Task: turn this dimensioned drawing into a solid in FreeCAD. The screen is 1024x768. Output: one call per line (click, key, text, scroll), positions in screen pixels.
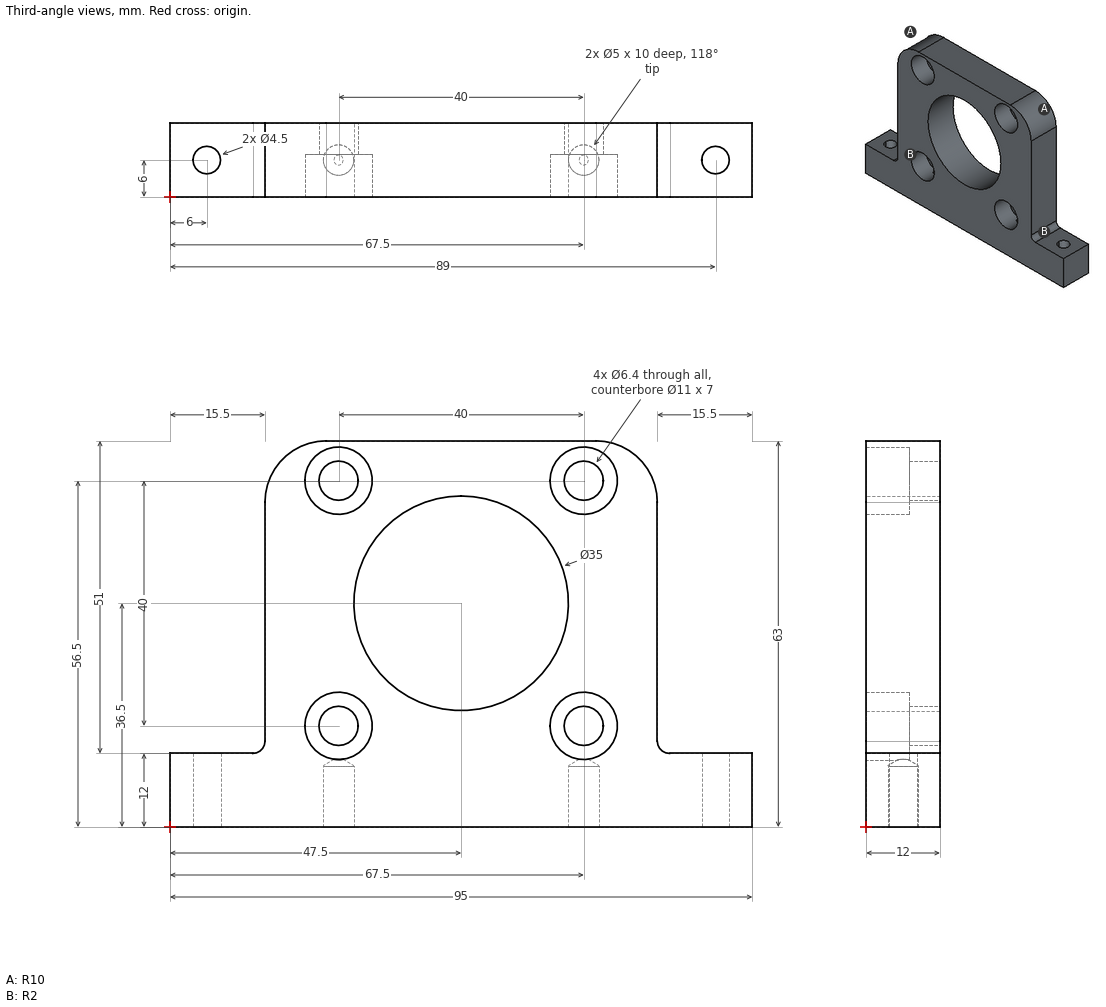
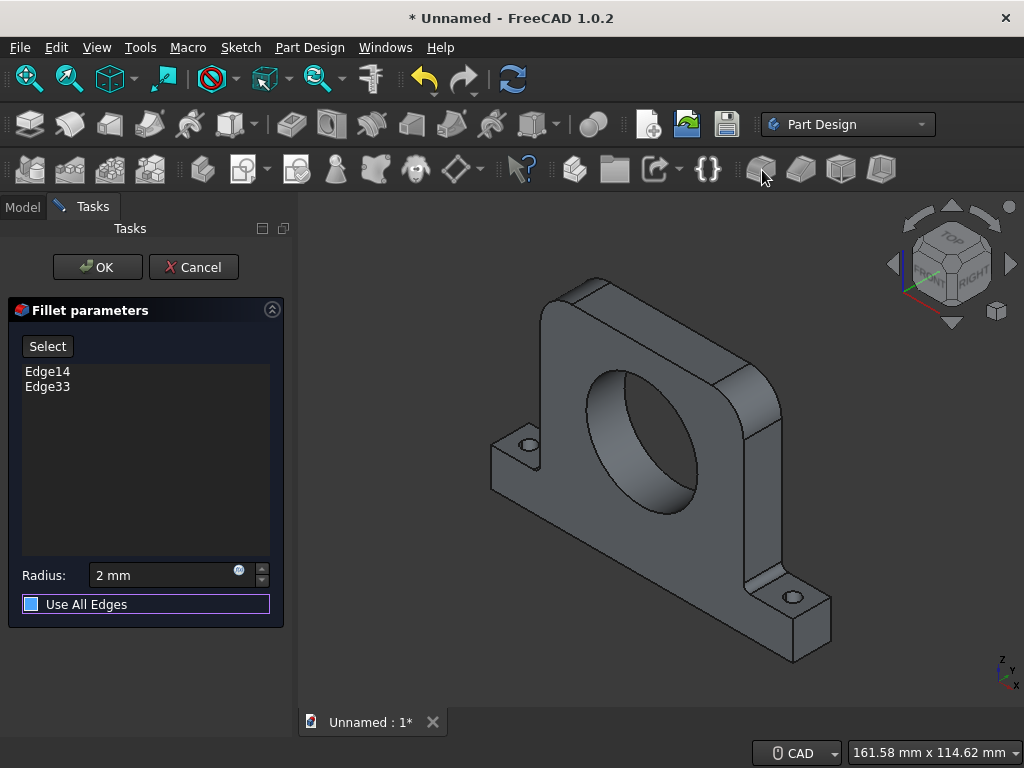
click(98, 267)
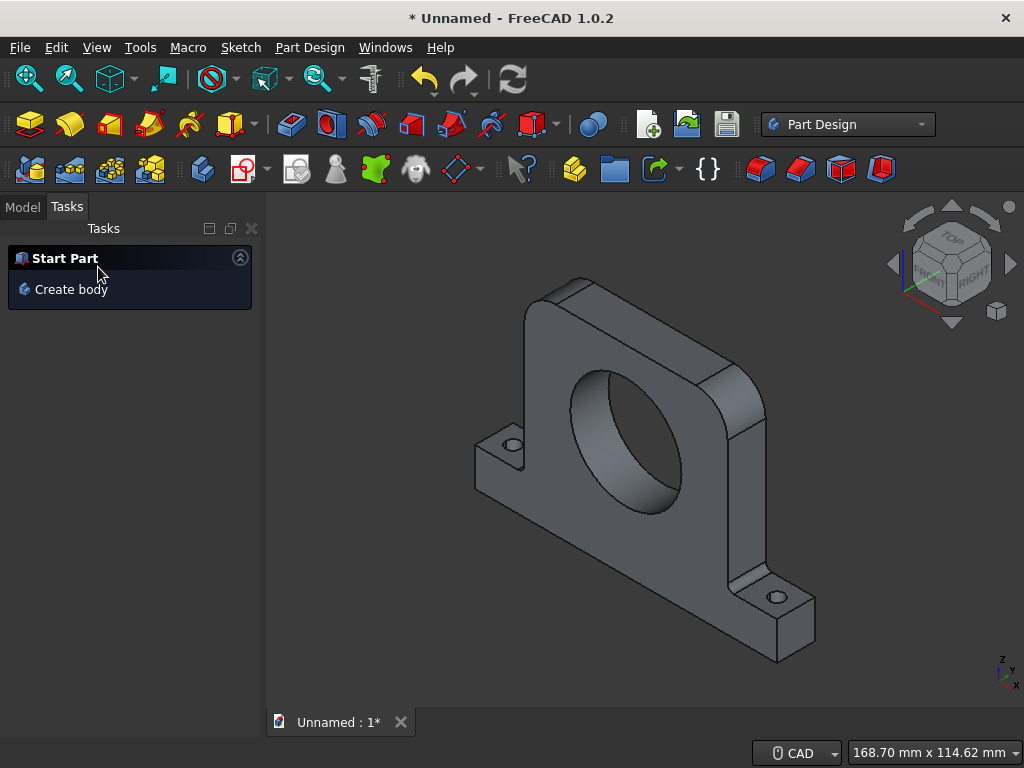
click(244, 170)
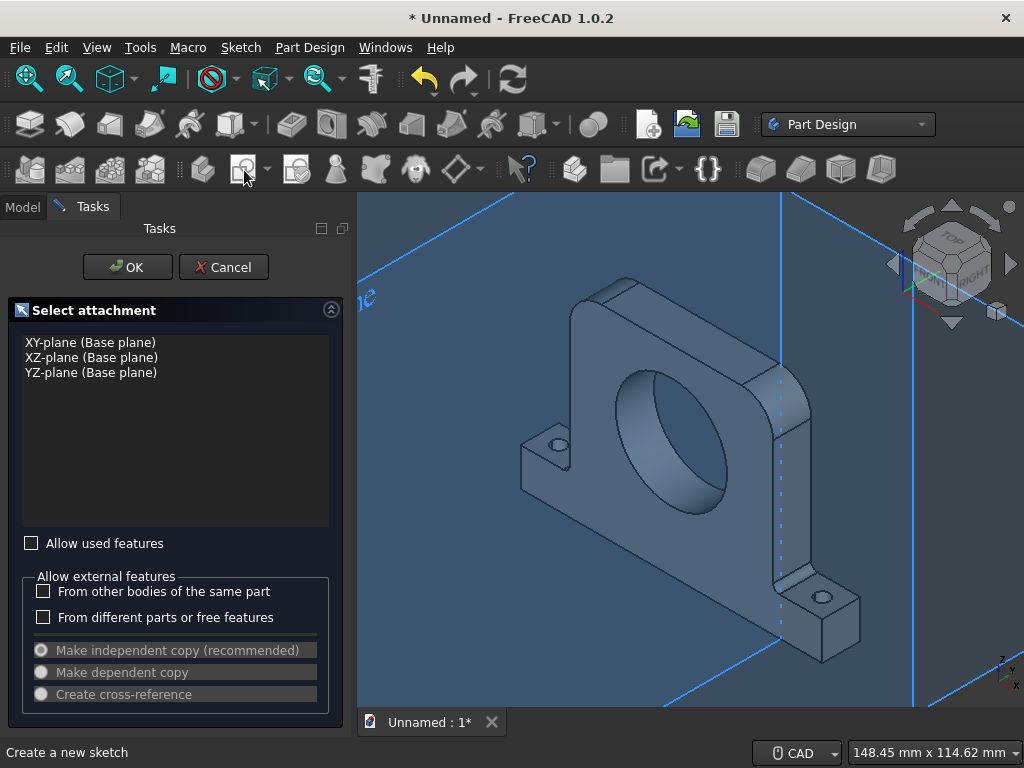
click(82, 358)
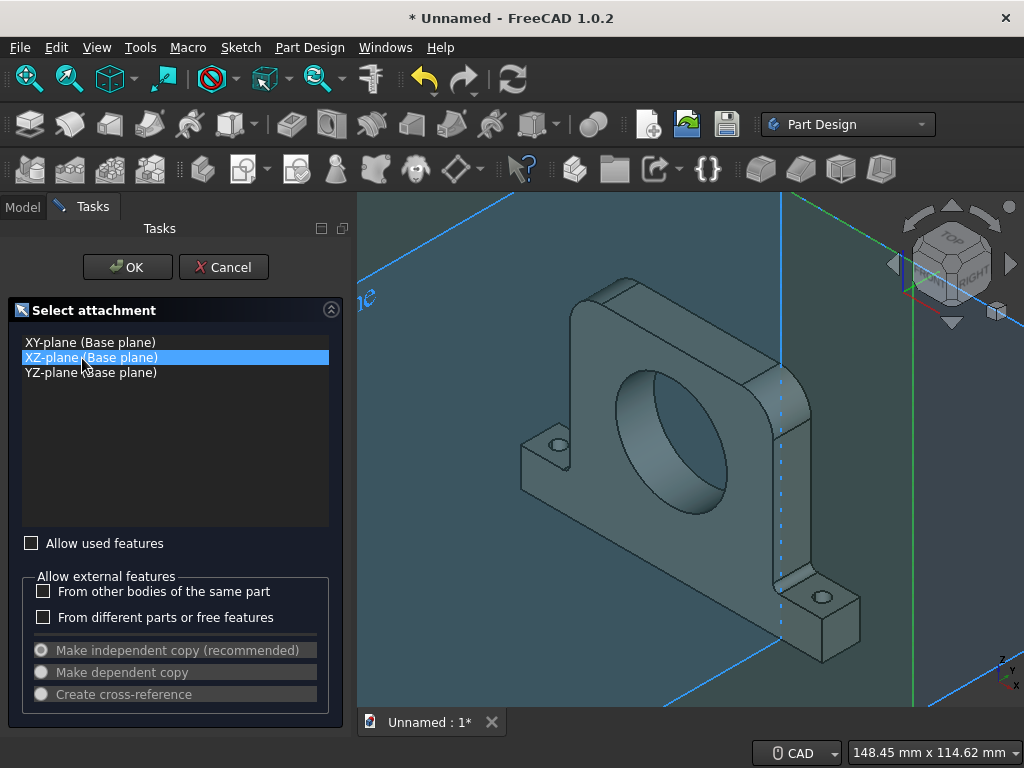
click(128, 267)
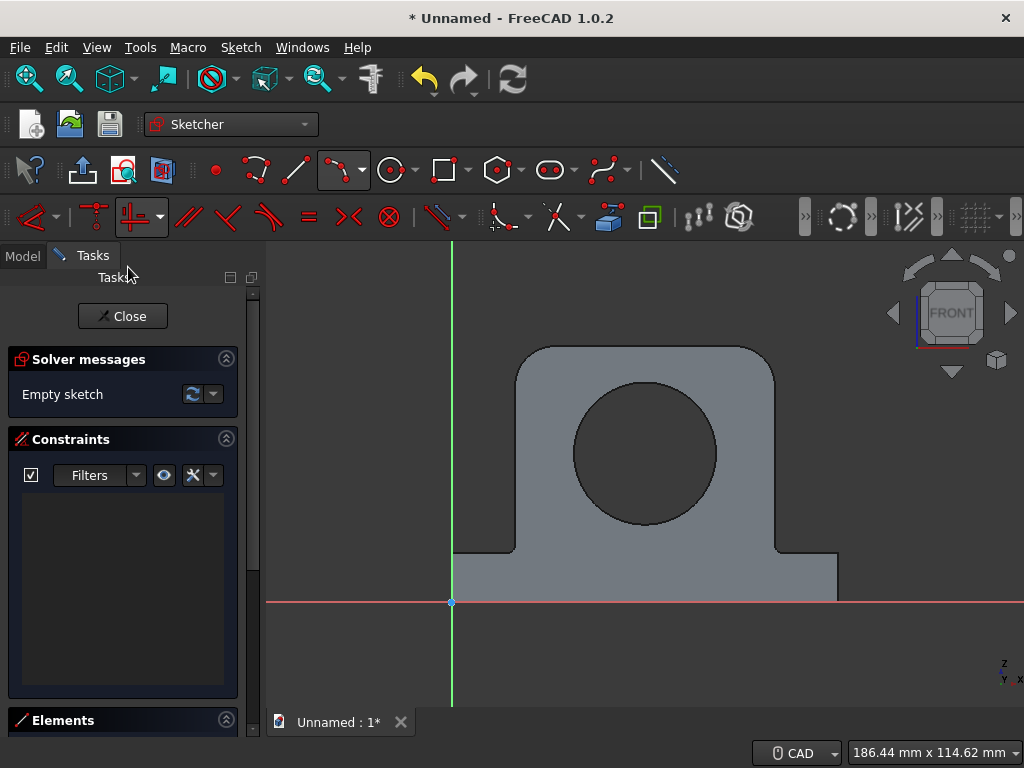
key(g)
key(c)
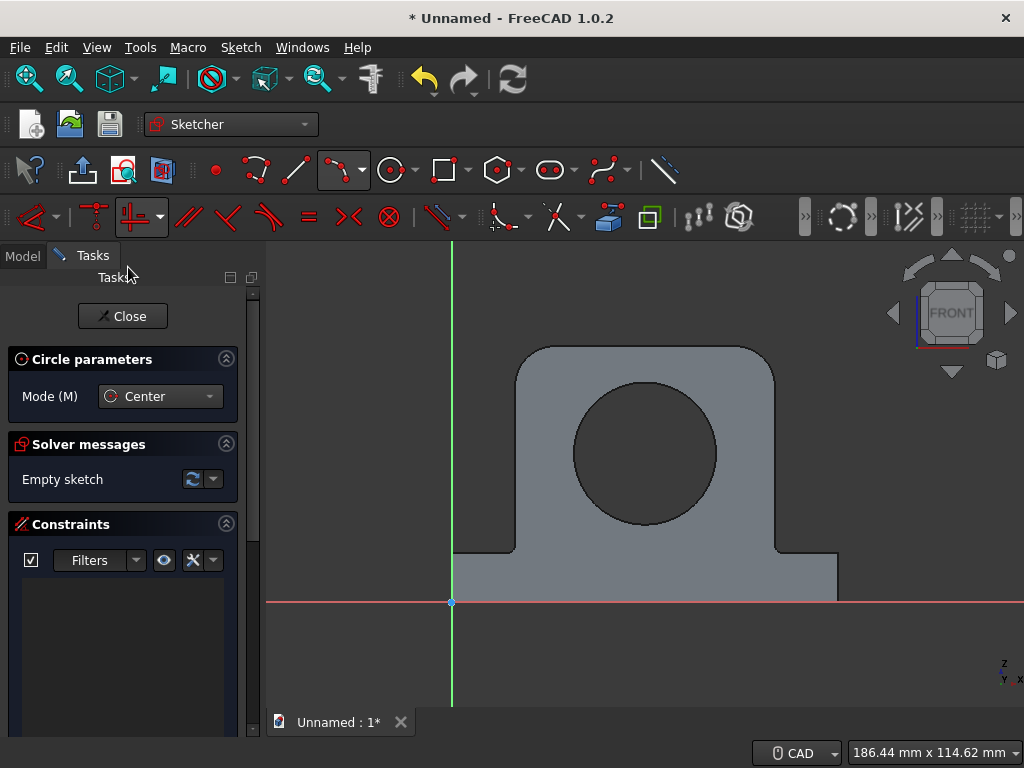
scroll(726, 372, up, 3)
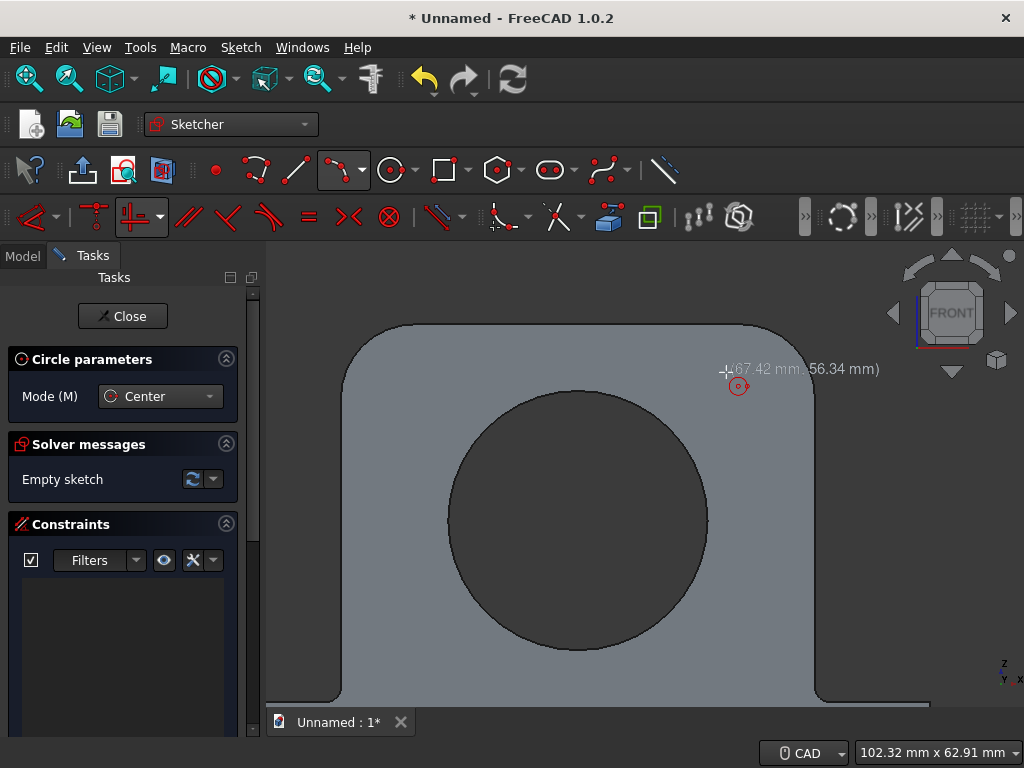
click(726, 372)
click(743, 356)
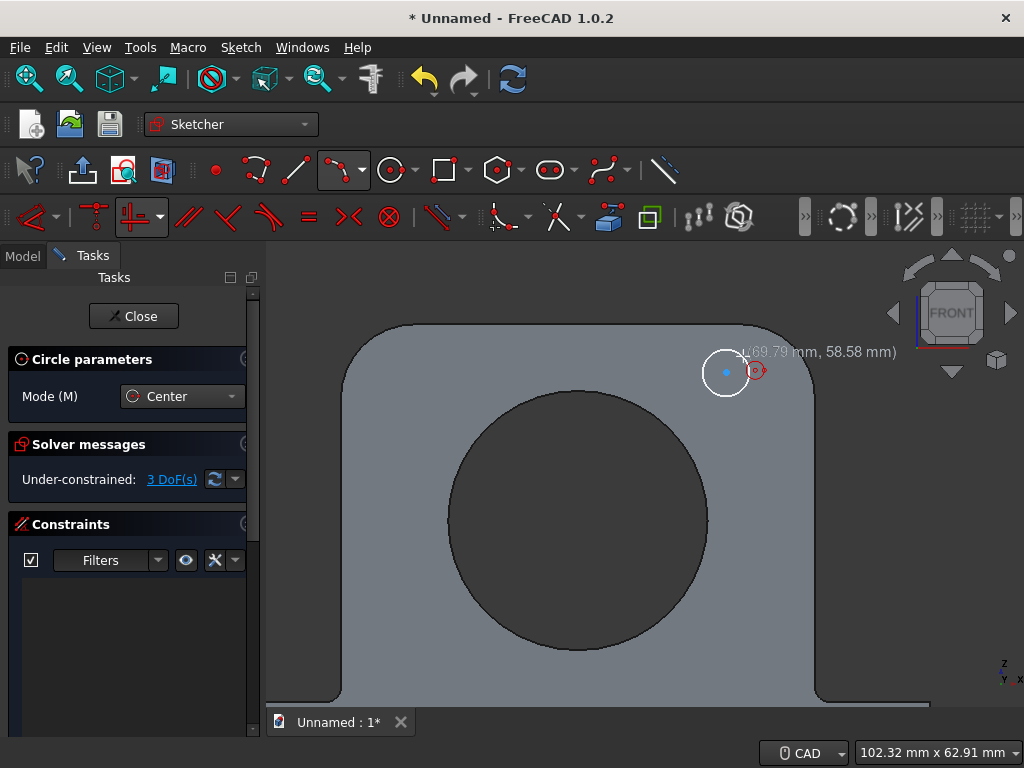
click(430, 372)
click(447, 356)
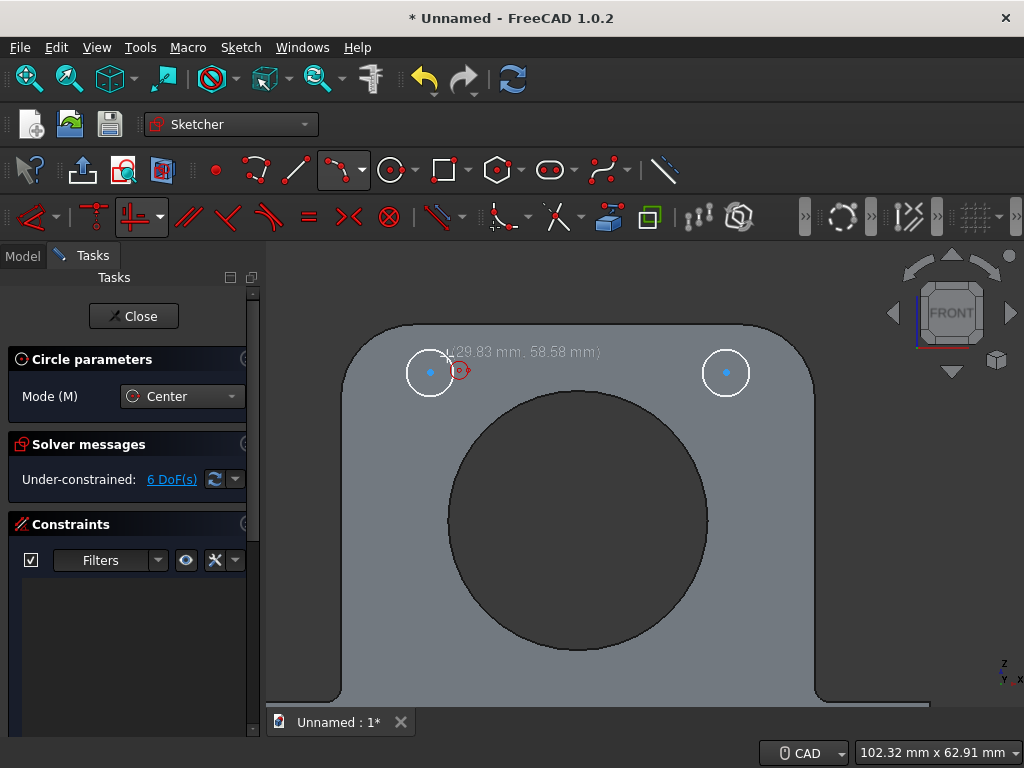
click(430, 669)
click(447, 652)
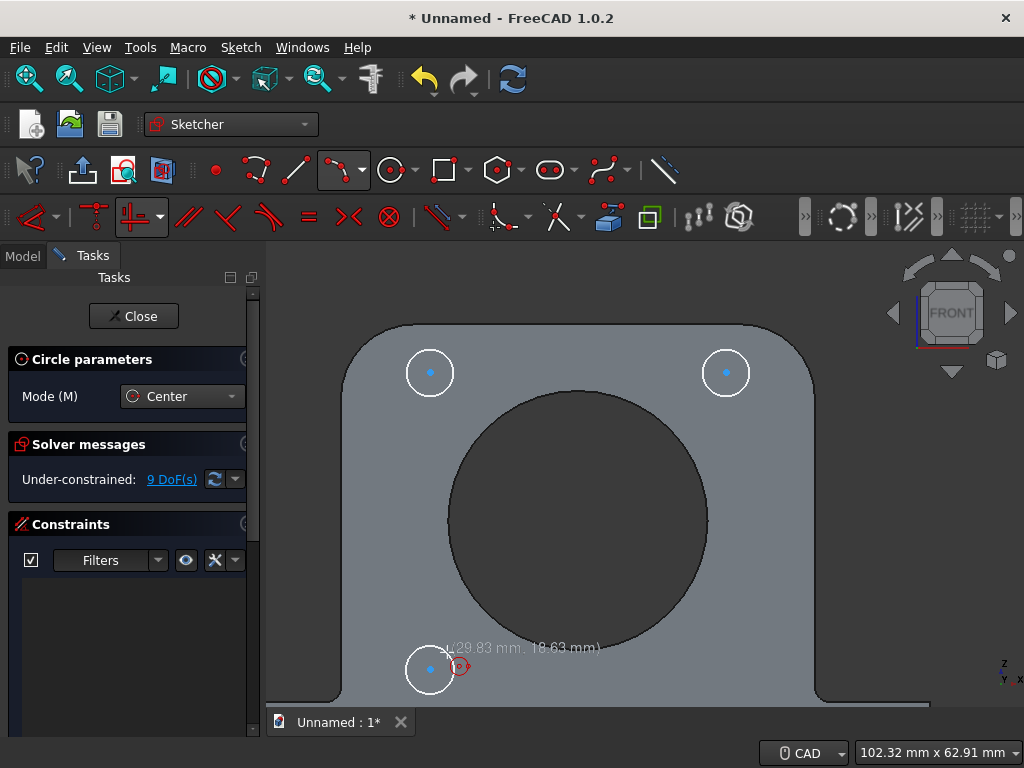
click(726, 669)
click(743, 652)
key(Escape)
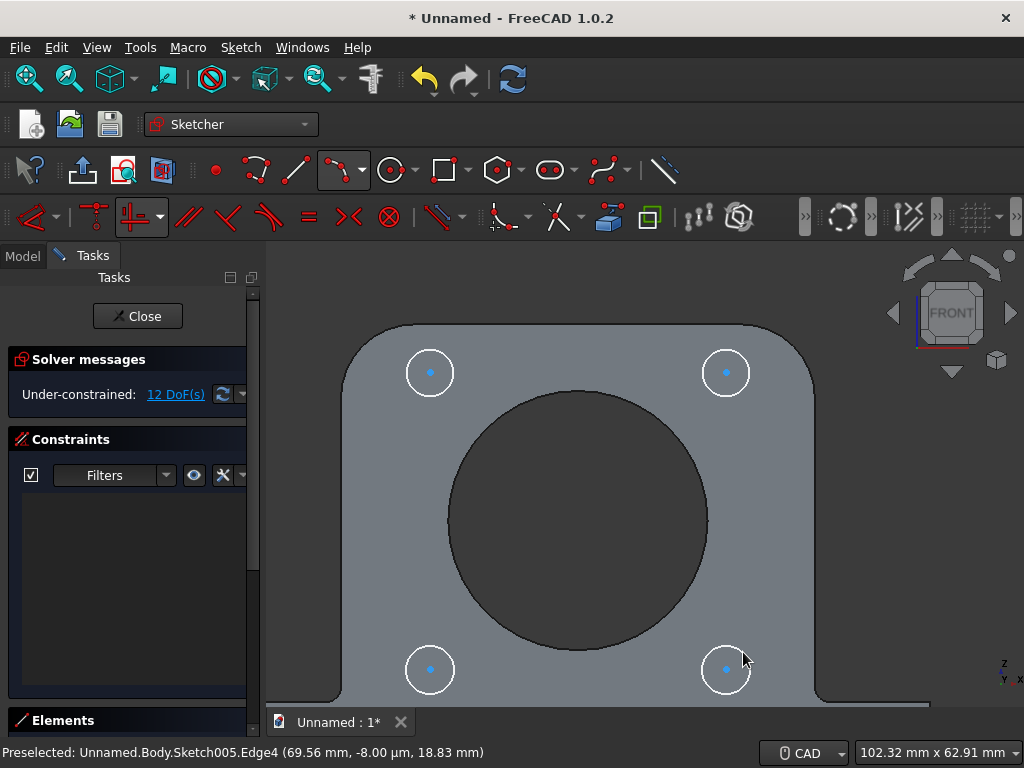
click(742, 356)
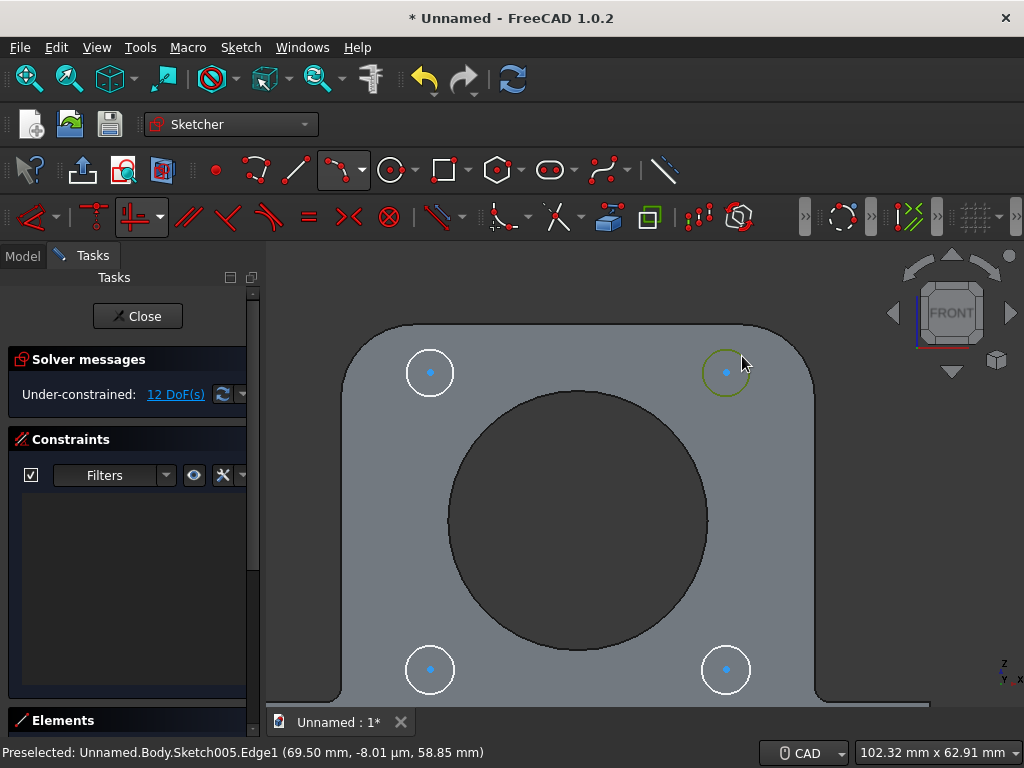
click(446, 356)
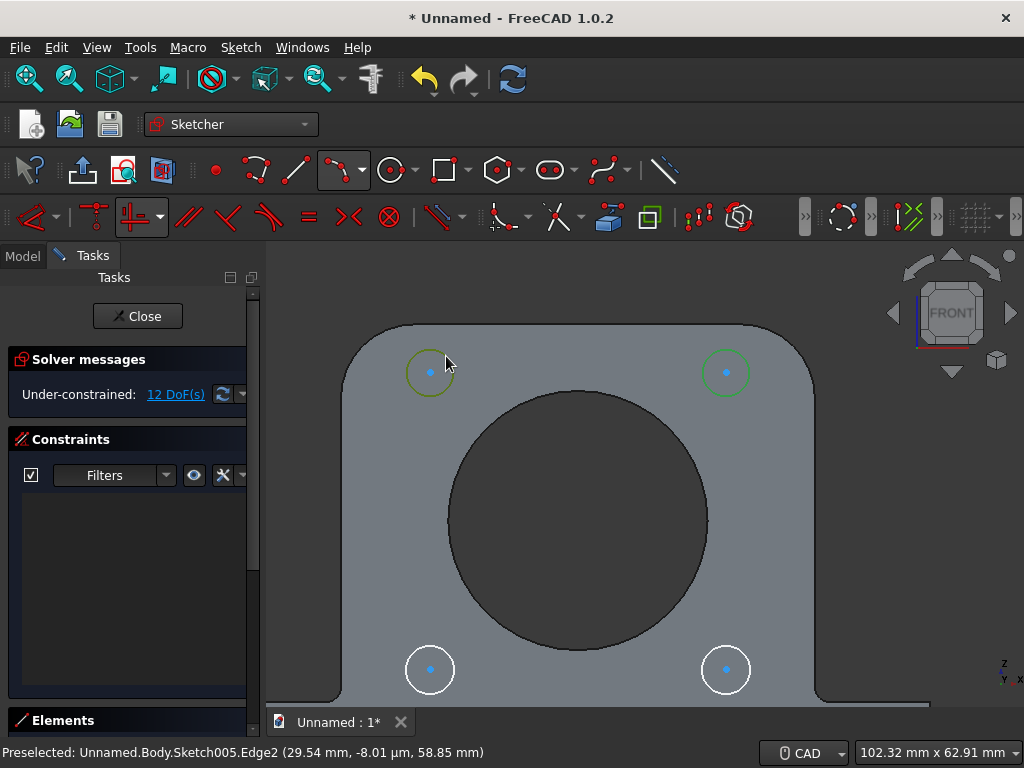
click(447, 653)